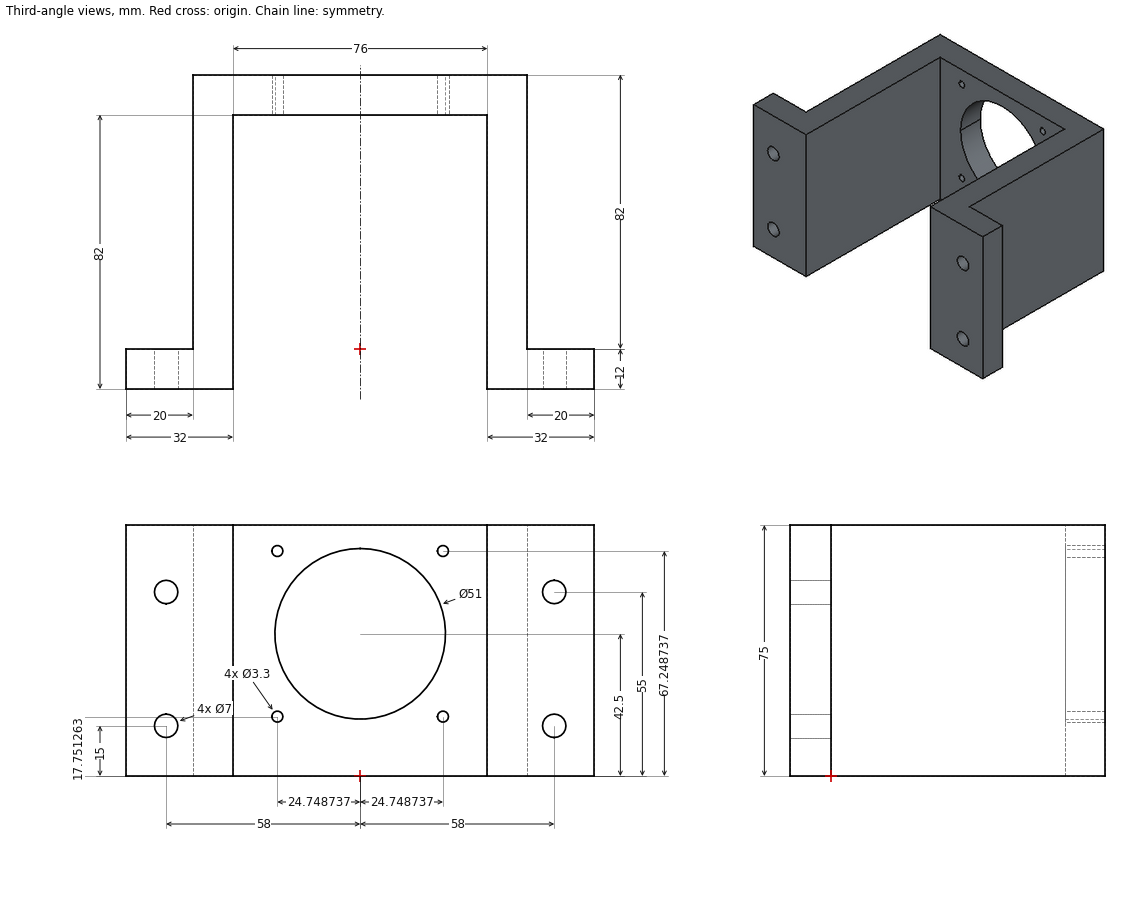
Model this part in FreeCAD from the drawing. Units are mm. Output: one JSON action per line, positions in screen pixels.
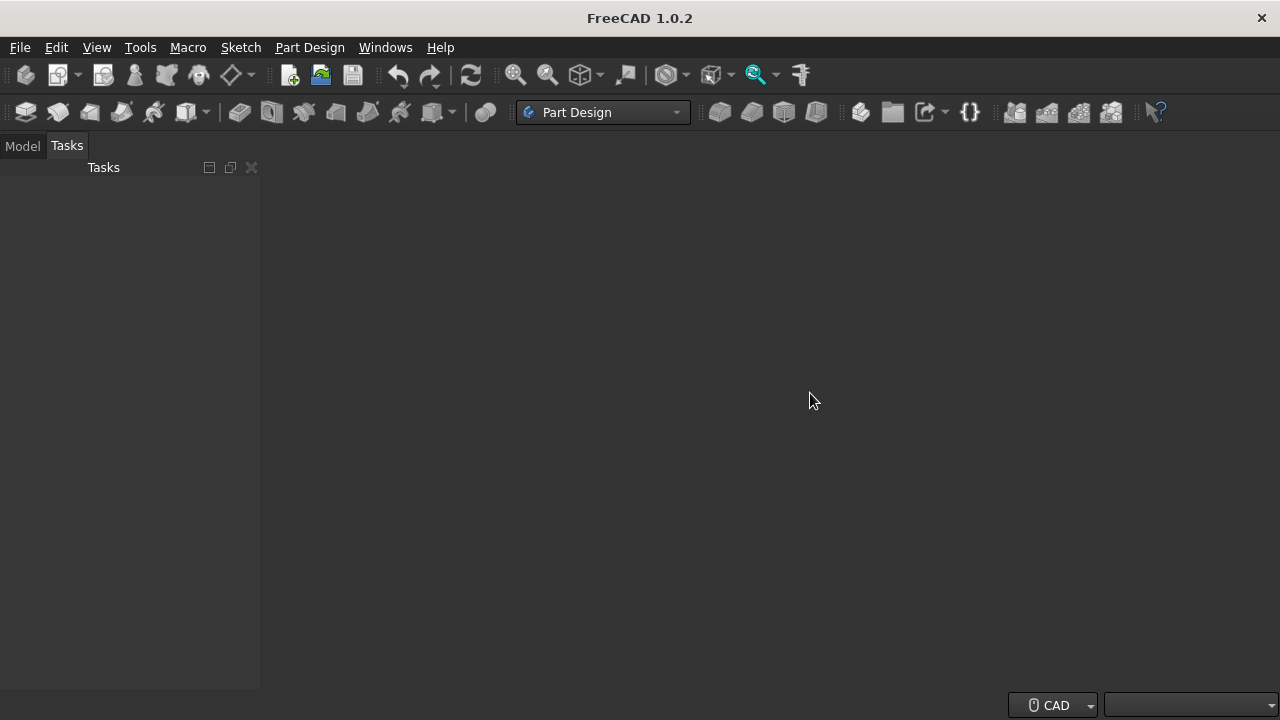
{"action": "left_click", "coordinate": [290, 76]}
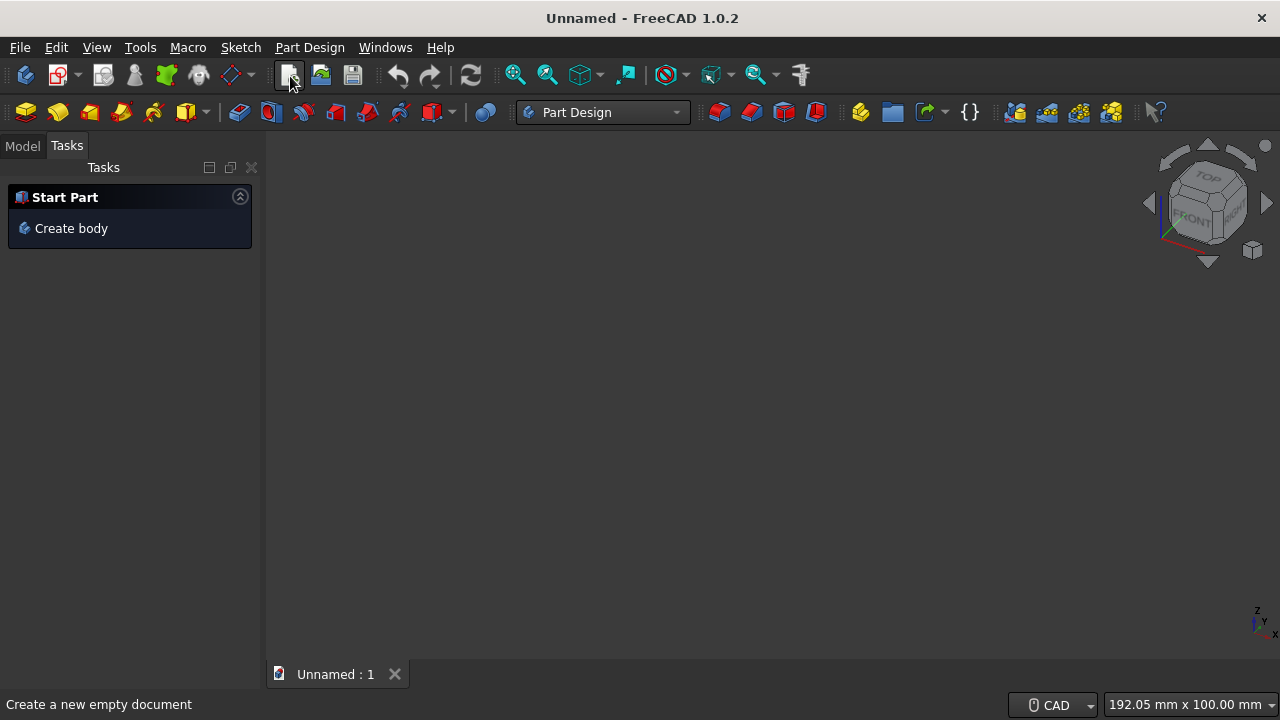
{"action": "left_click", "coordinate": [58, 76]}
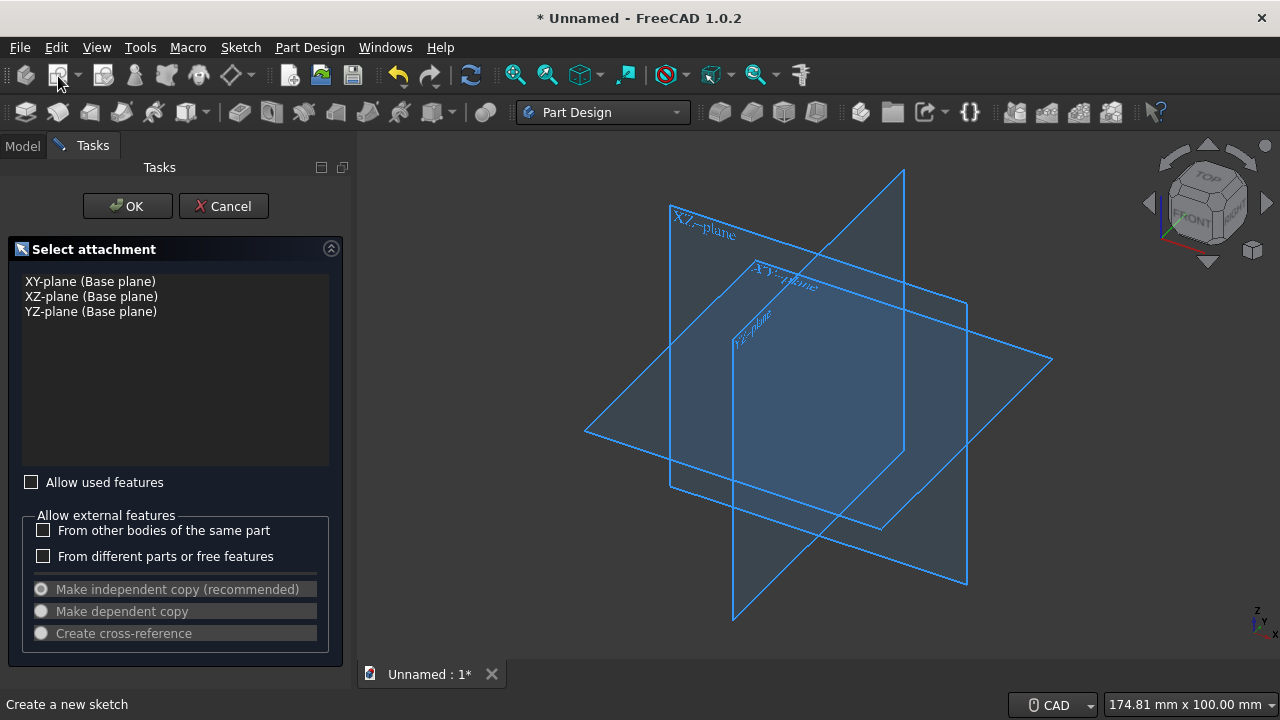
{"action": "left_click", "coordinate": [82, 282]}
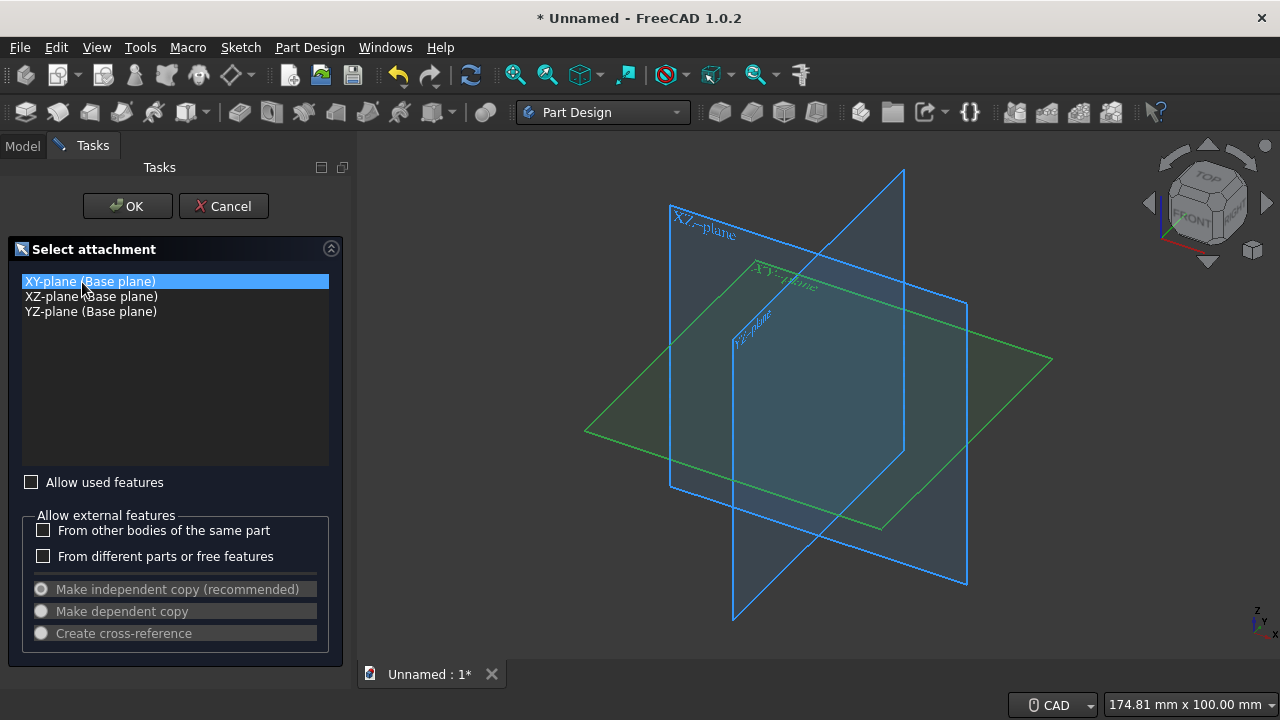
{"action": "left_click", "coordinate": [128, 206]}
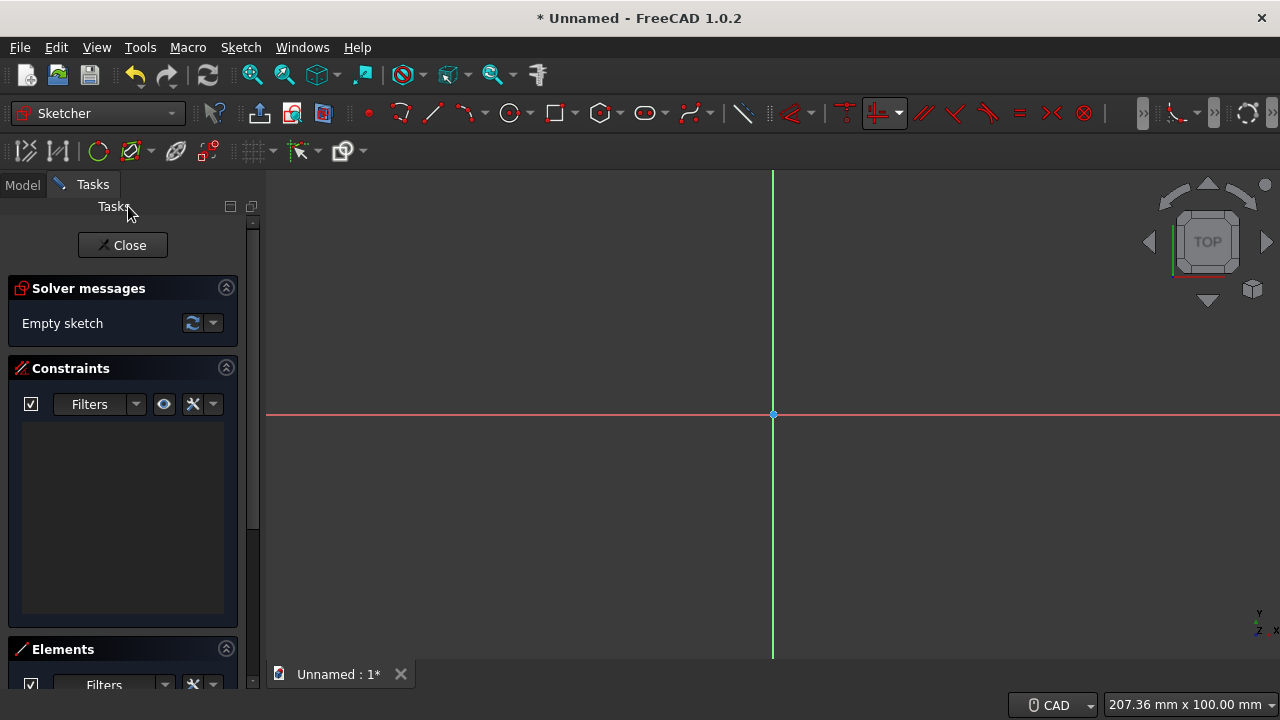
{"action": "scroll", "coordinate": [621, 623], "scroll_direction": "down", "scroll_amount": 3}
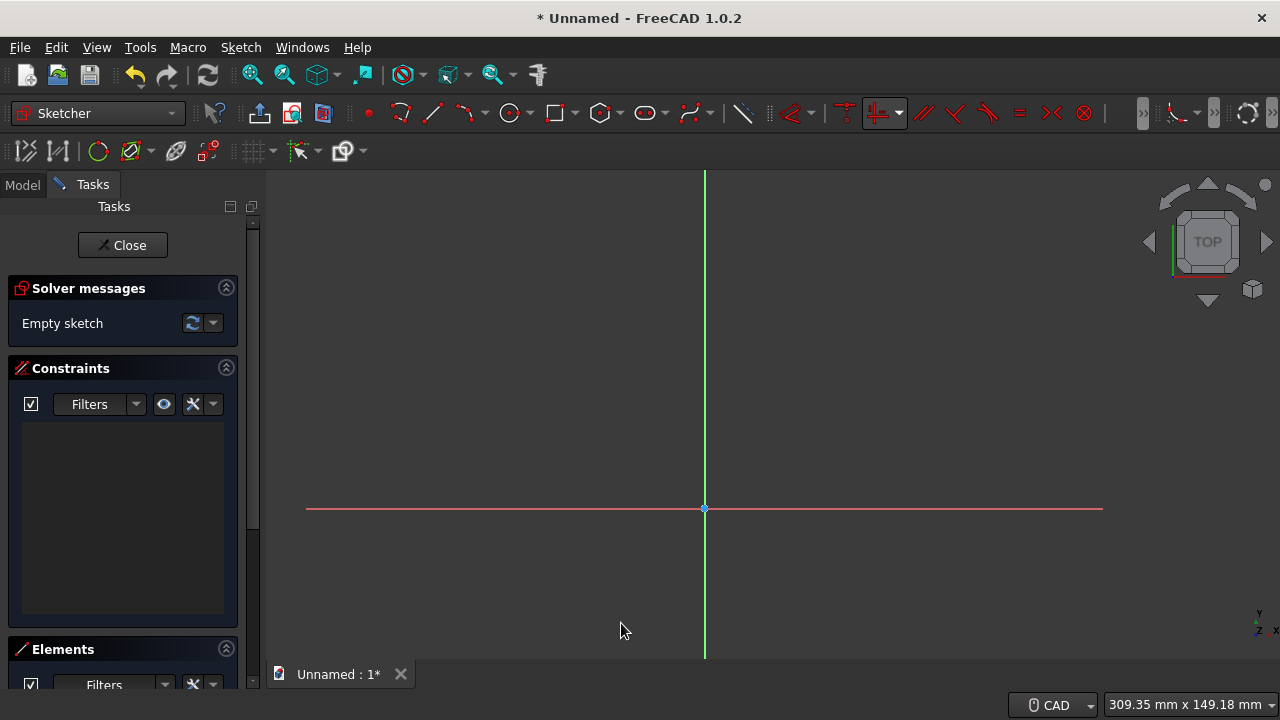
{"action": "left_click", "coordinate": [402, 114]}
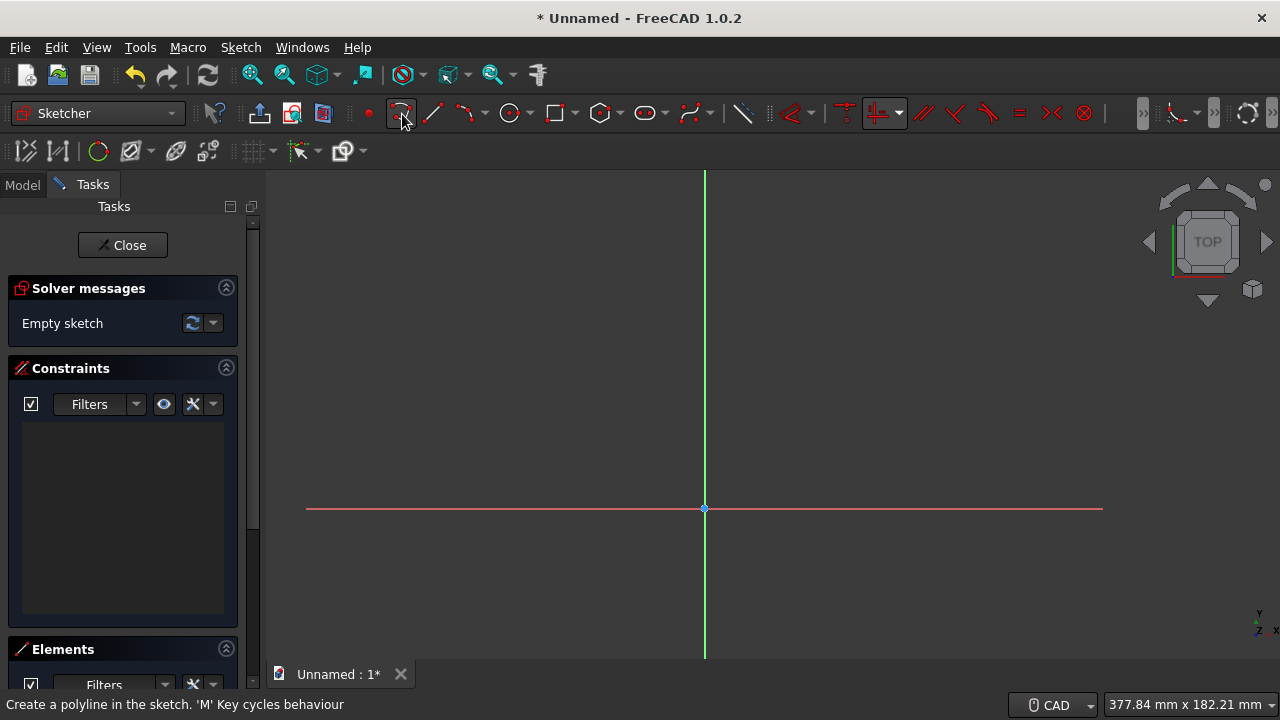
{"action": "left_click", "coordinate": [603, 541]}
{"action": "left_click", "coordinate": [603, 321]}
{"action": "left_click", "coordinate": [807, 321]}
{"action": "left_click", "coordinate": [807, 541]}
{"action": "left_click", "coordinate": [892, 541]}
{"action": "left_click", "coordinate": [892, 509]}
{"action": "left_click", "coordinate": [839, 500]}
{"action": "left_click", "coordinate": [839, 289]}
{"action": "left_click", "coordinate": [570, 289]}
{"action": "left_click", "coordinate": [570, 509]}
{"action": "left_click", "coordinate": [517, 500]}
{"action": "left_click", "coordinate": [517, 541]}
{"action": "left_click", "coordinate": [603, 542]}
{"action": "key", "text": "Escape"}
{"action": "key", "text": "Escape"}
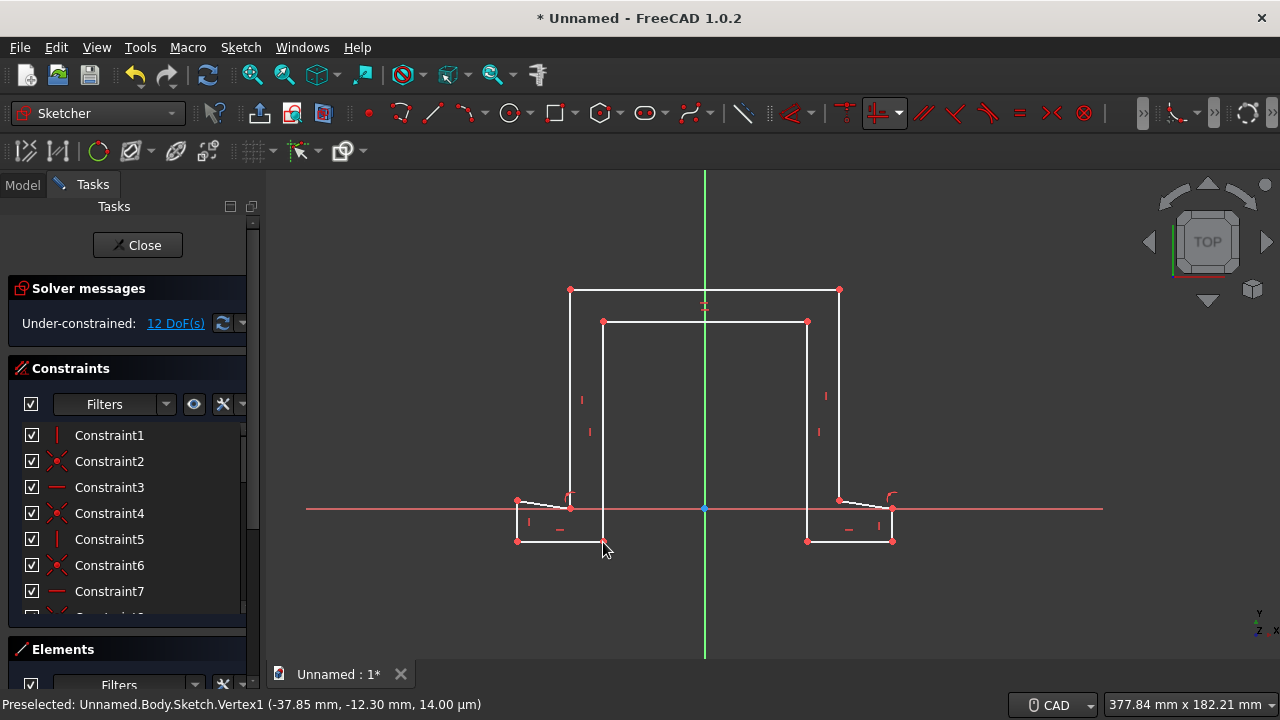
{"action": "left_click", "coordinate": [876, 507]}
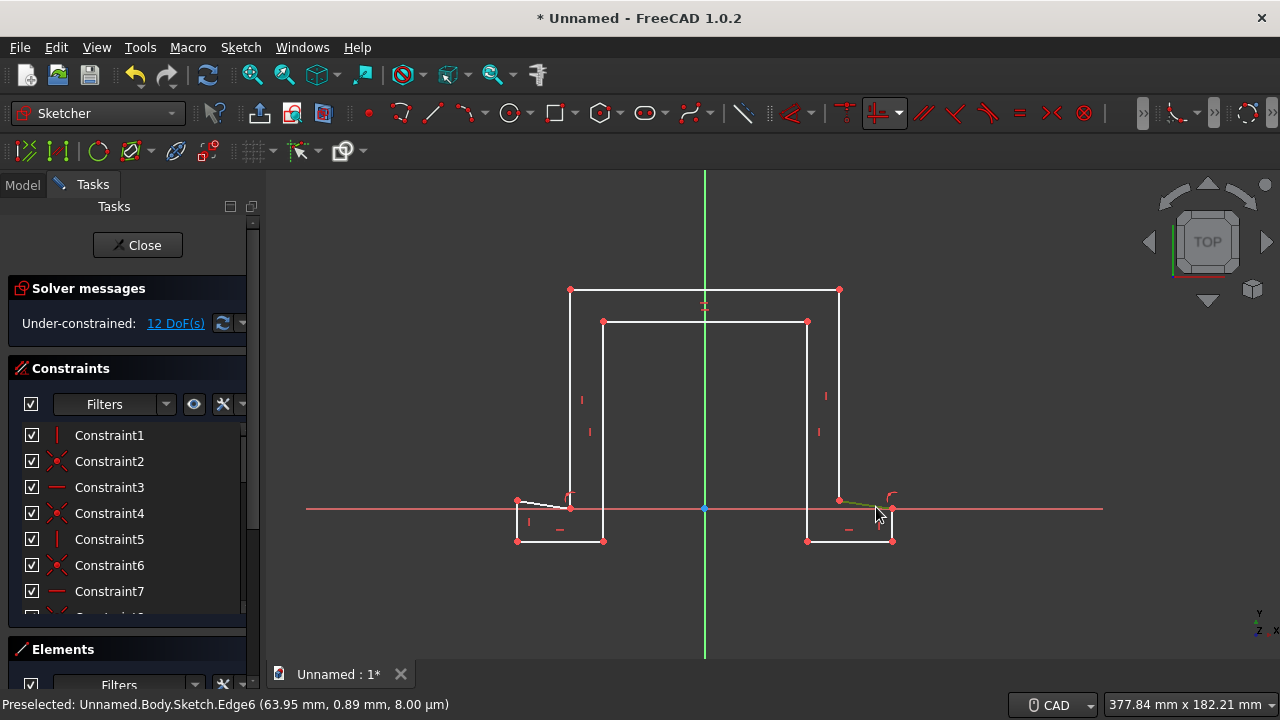
{"action": "left_click", "coordinate": [902, 114]}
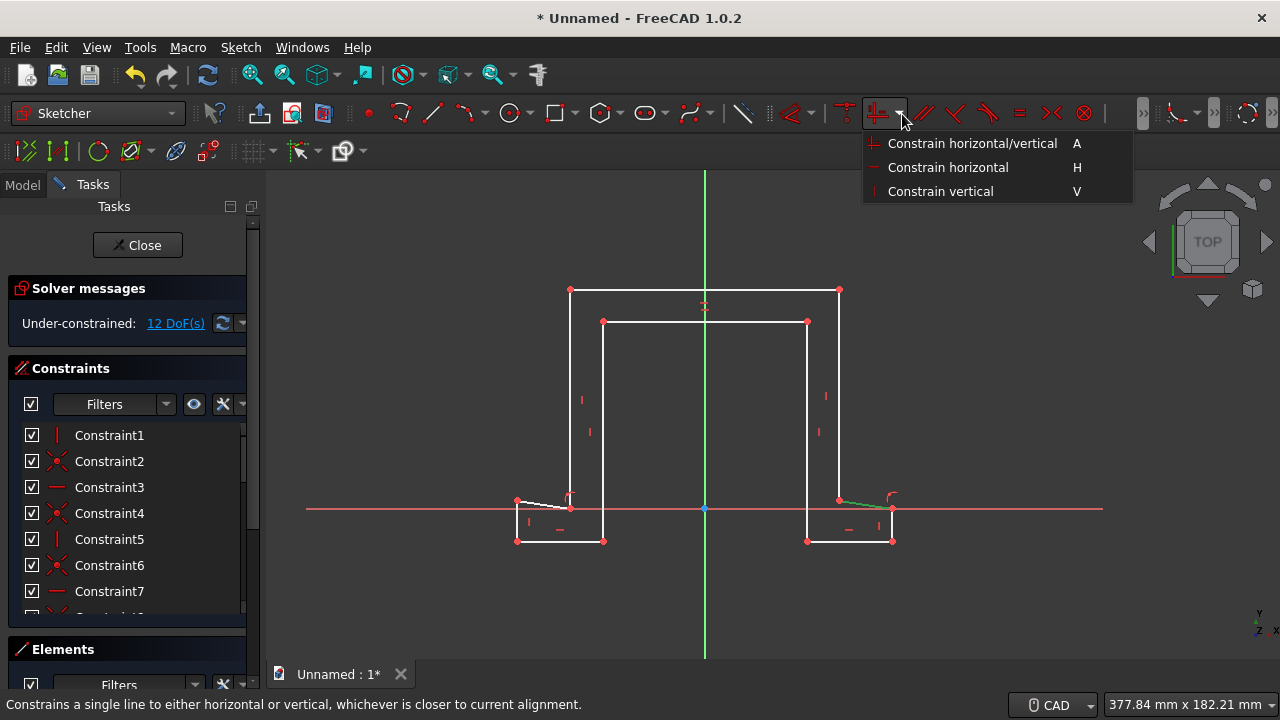
{"action": "left_click", "coordinate": [998, 167]}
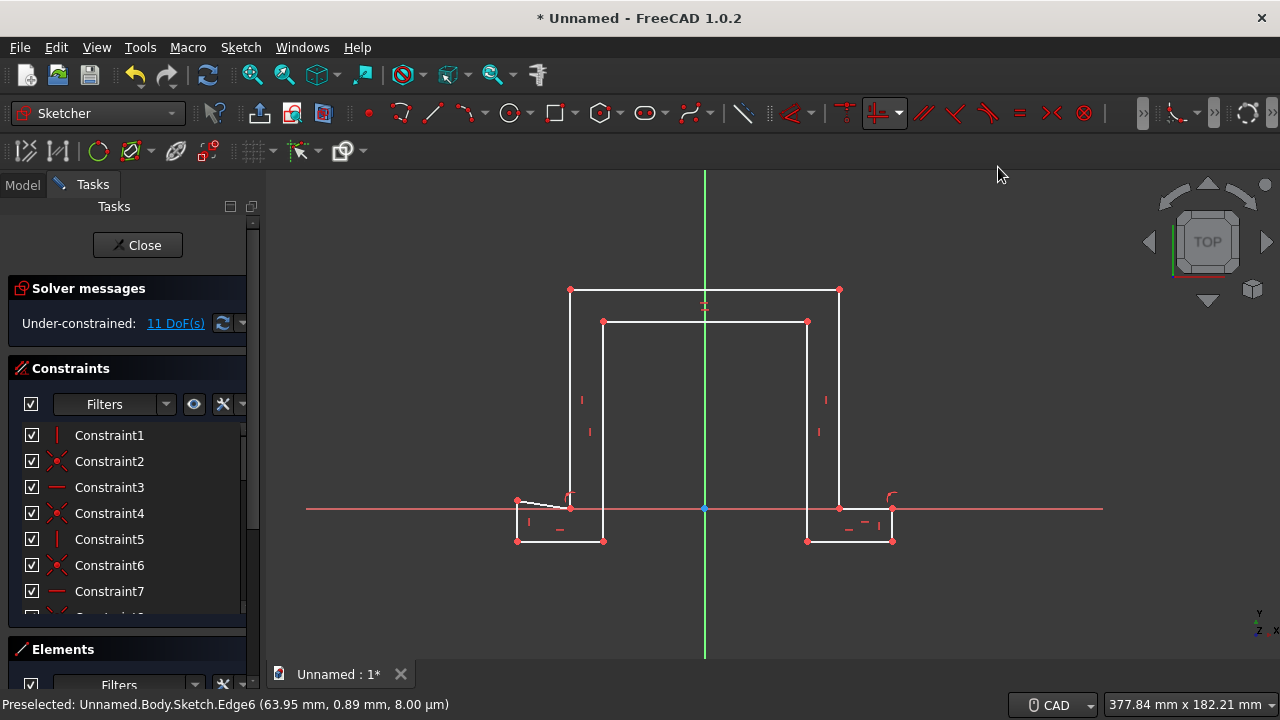
{"action": "left_click", "coordinate": [554, 507]}